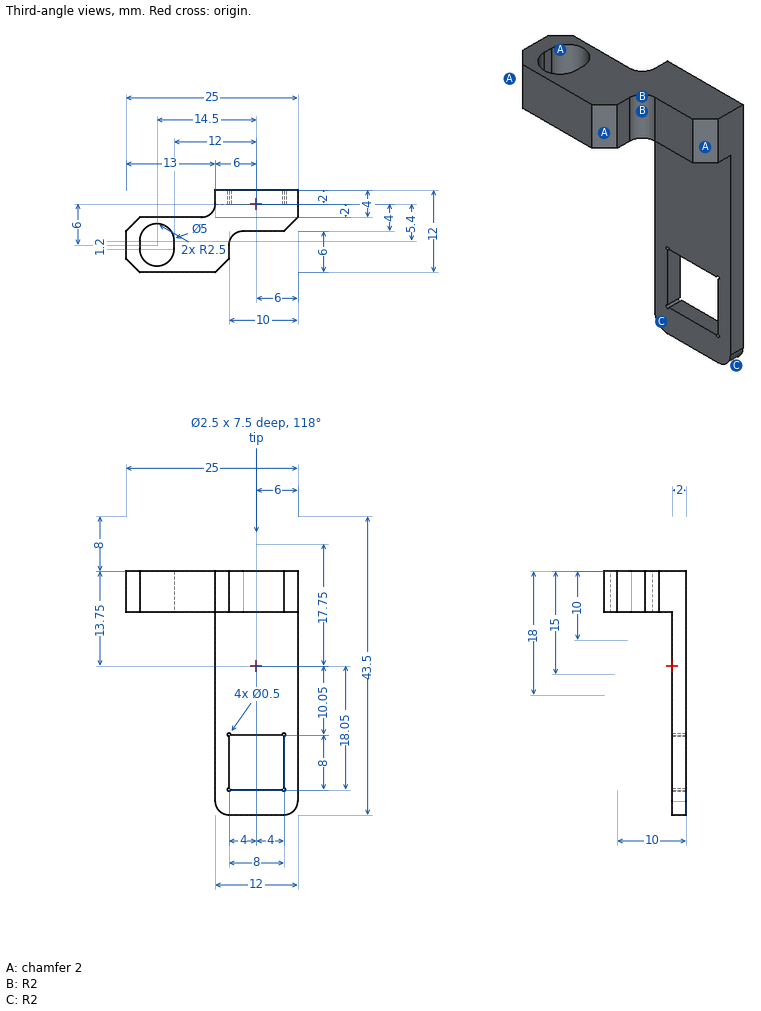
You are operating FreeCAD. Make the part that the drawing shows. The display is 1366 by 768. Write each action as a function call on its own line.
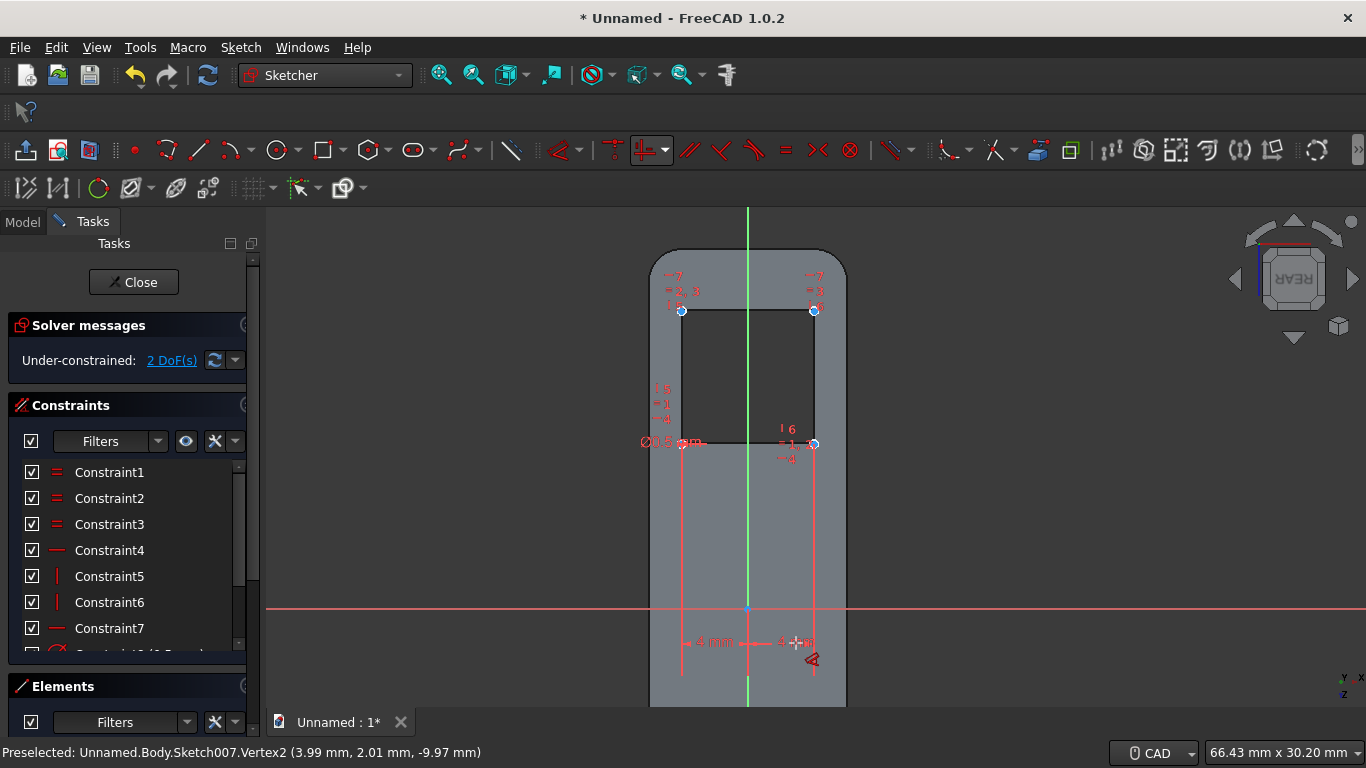
click(682, 444)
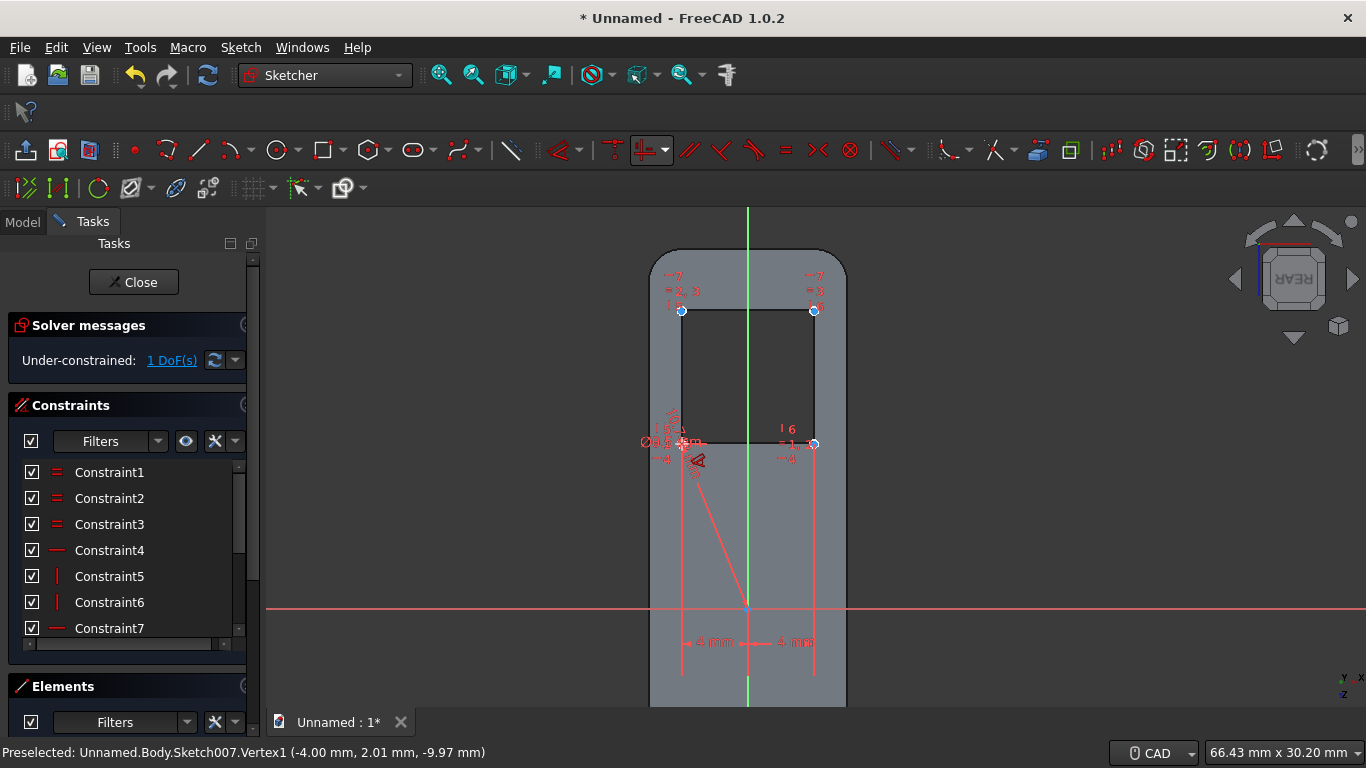
click(682, 311)
click(648, 378)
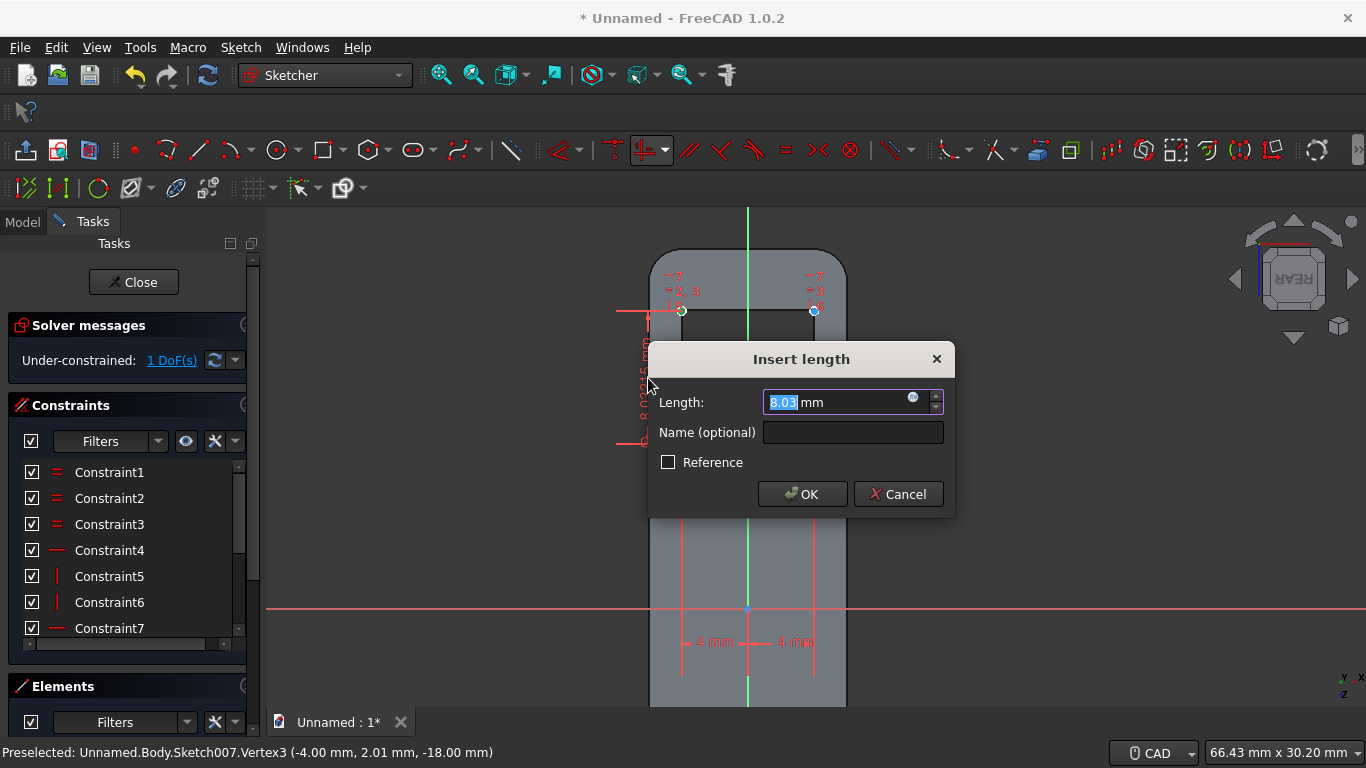
text(8)
key(Return)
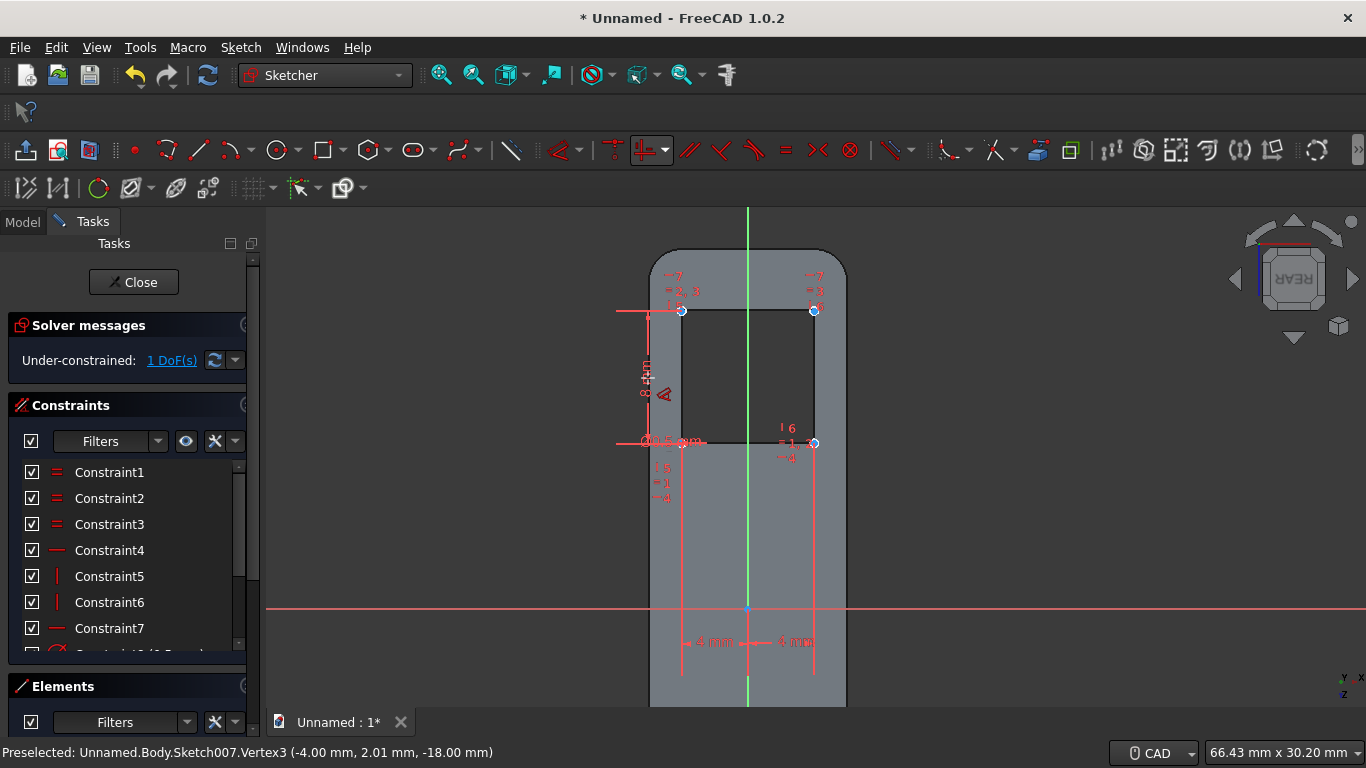
click(682, 444)
click(648, 526)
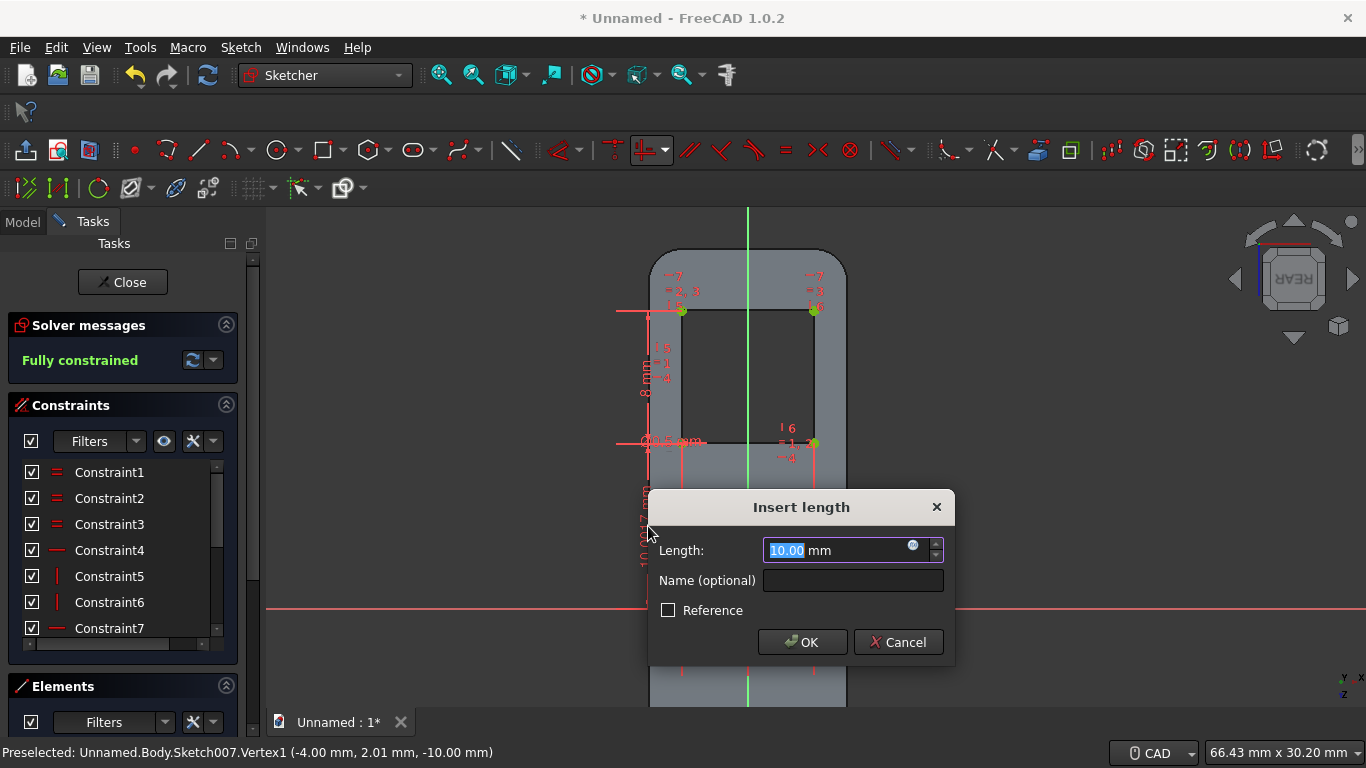
text(10.05)
key(Return)
key(Escape)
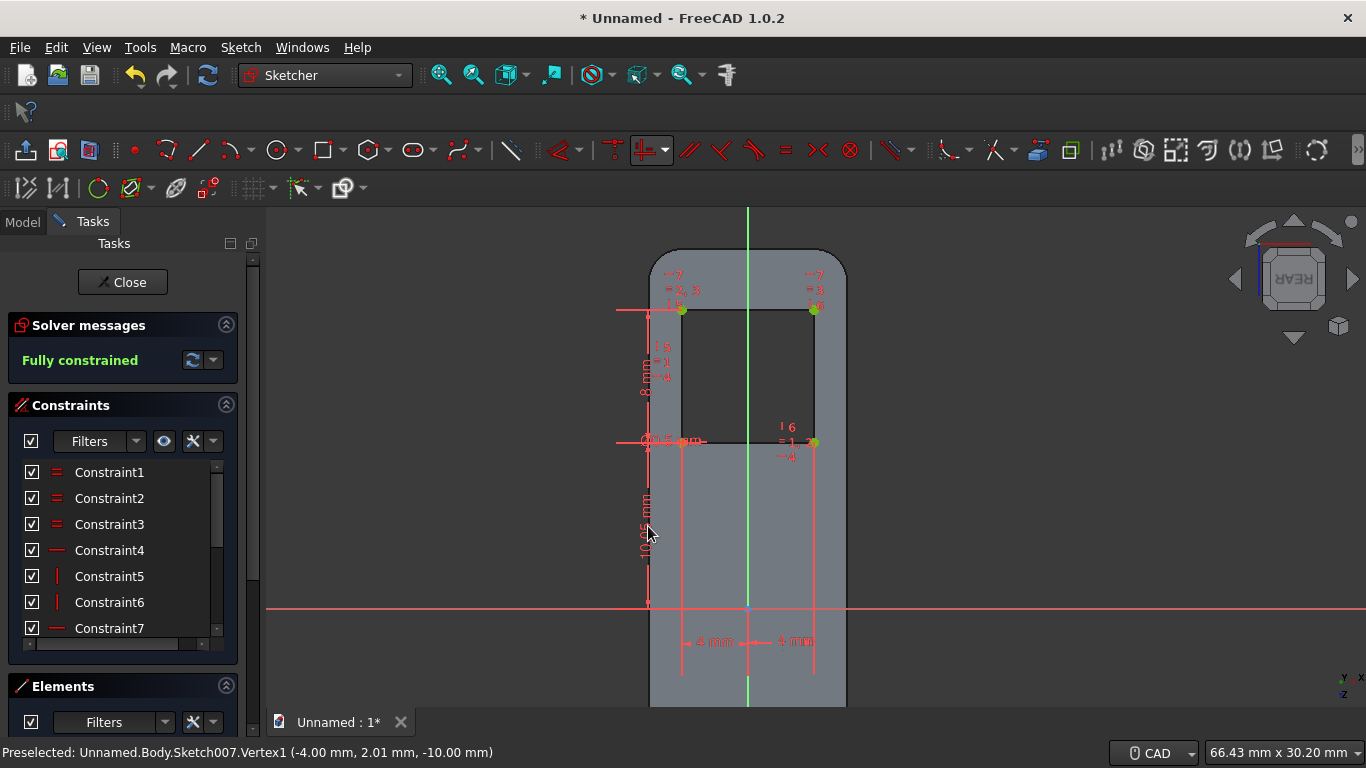
click(123, 282)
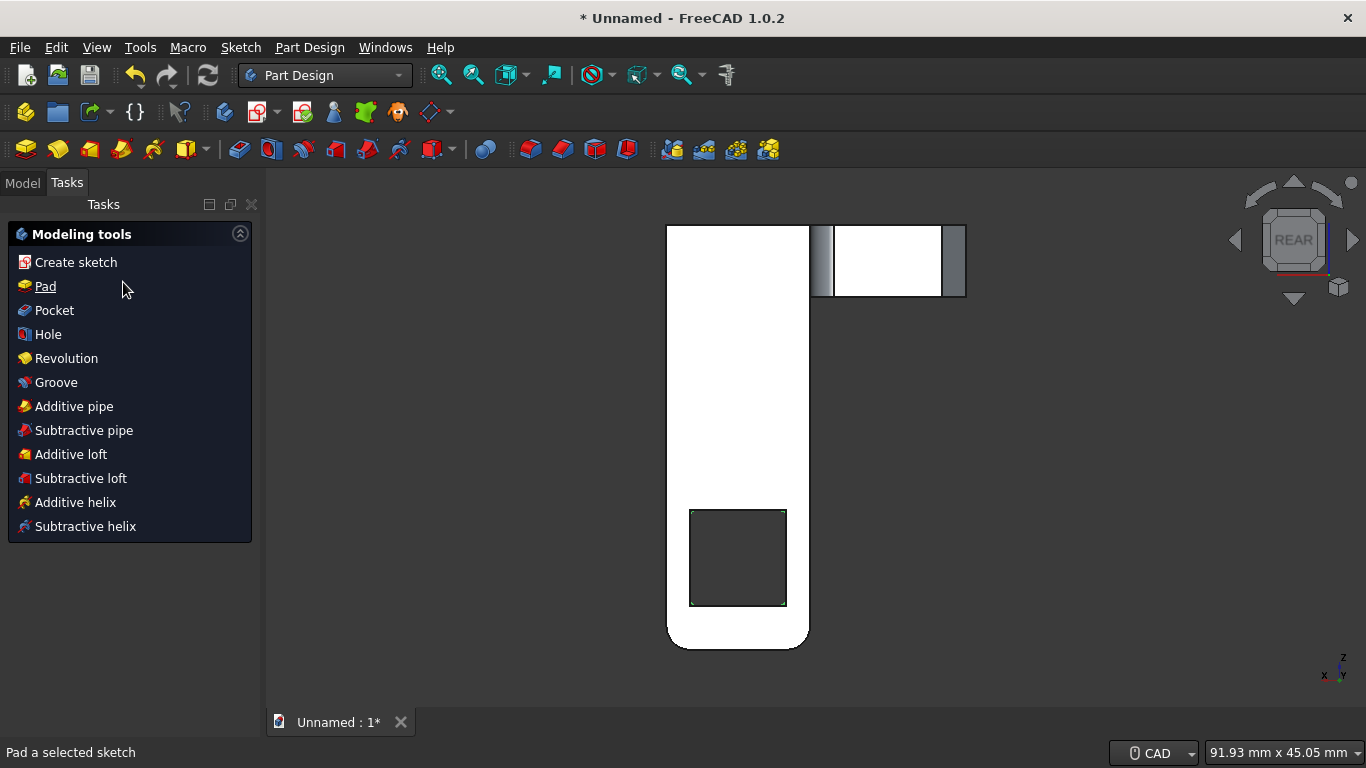
click(240, 150)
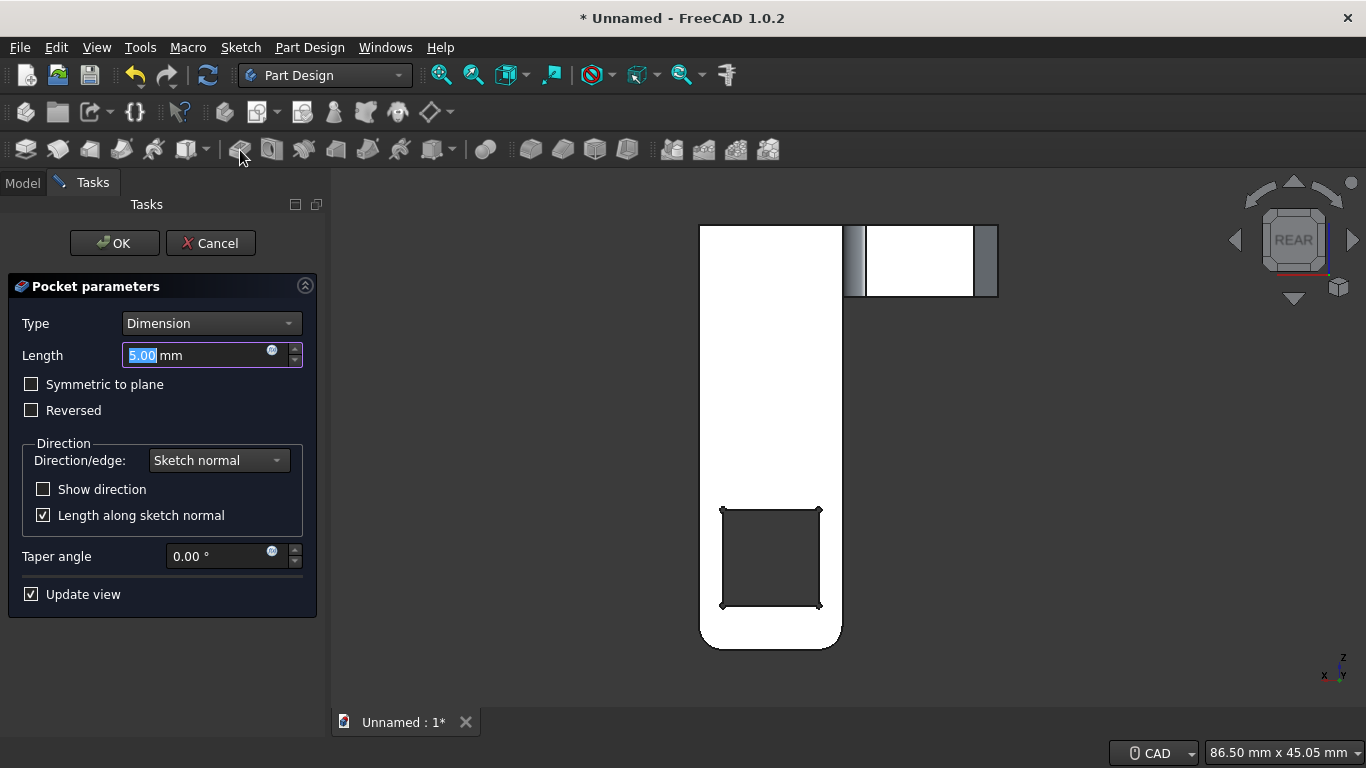
text(10)
key(Tab)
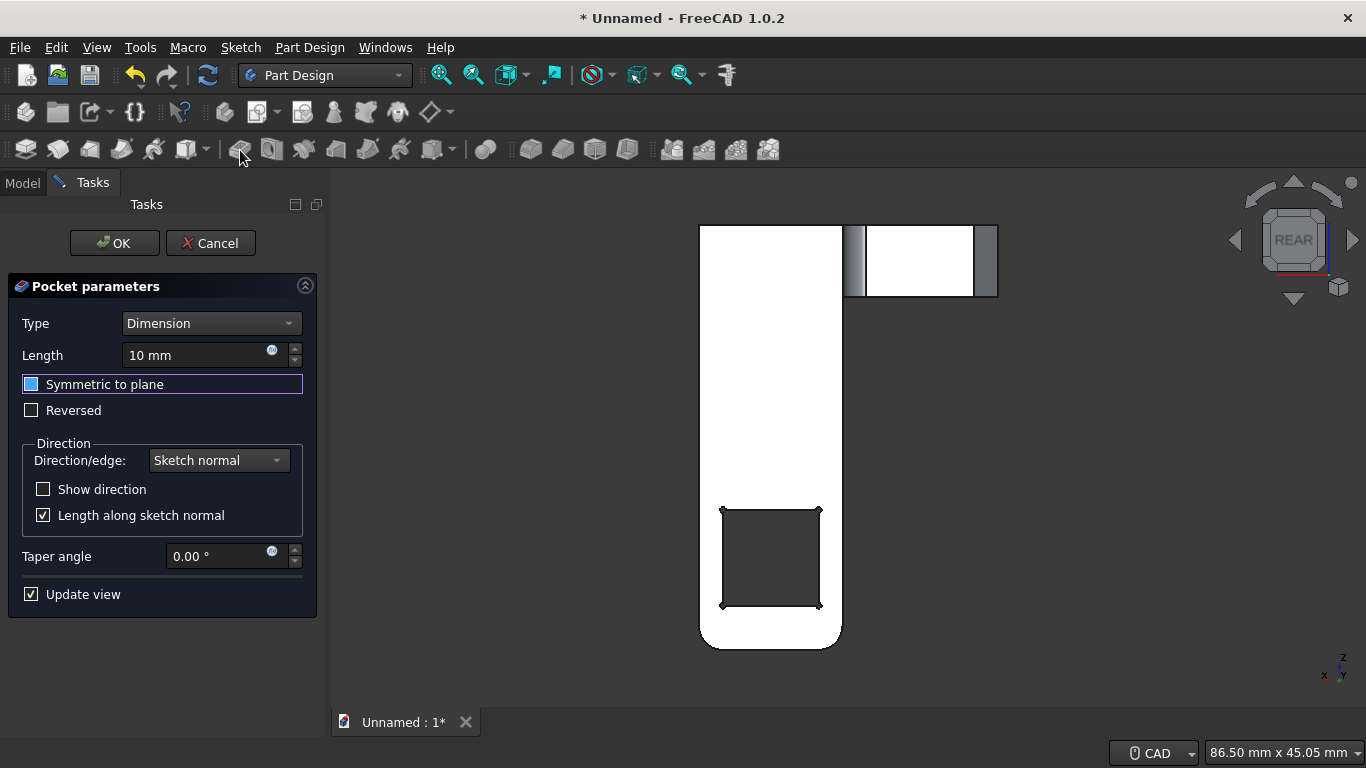
click(115, 243)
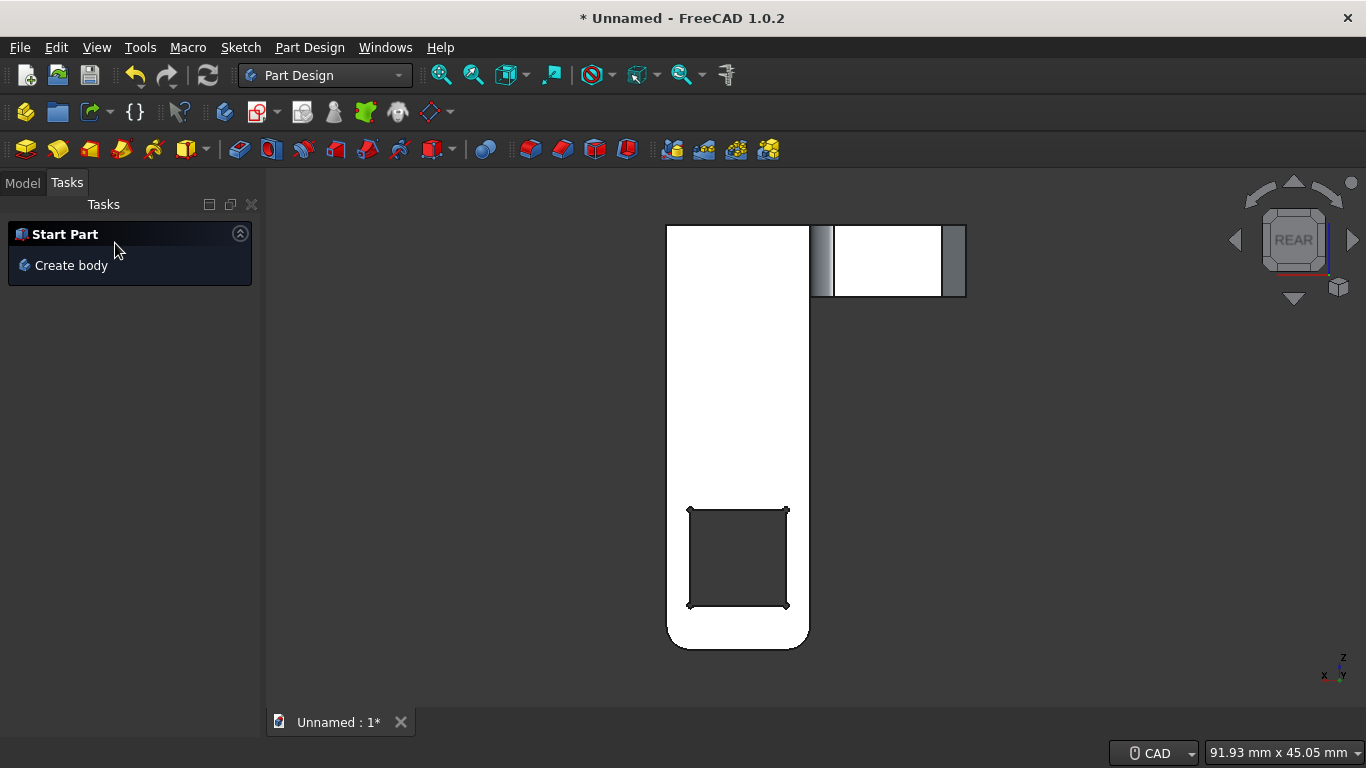
key(0)